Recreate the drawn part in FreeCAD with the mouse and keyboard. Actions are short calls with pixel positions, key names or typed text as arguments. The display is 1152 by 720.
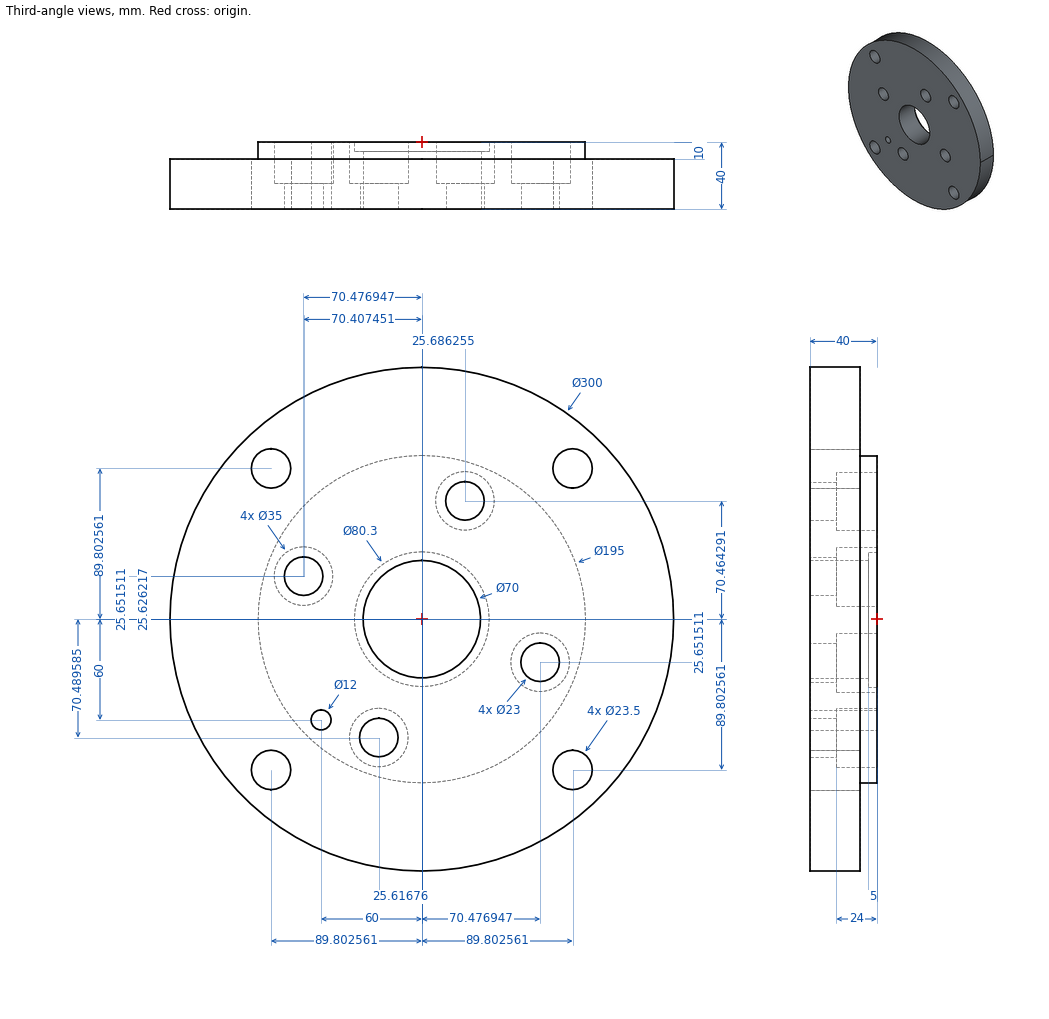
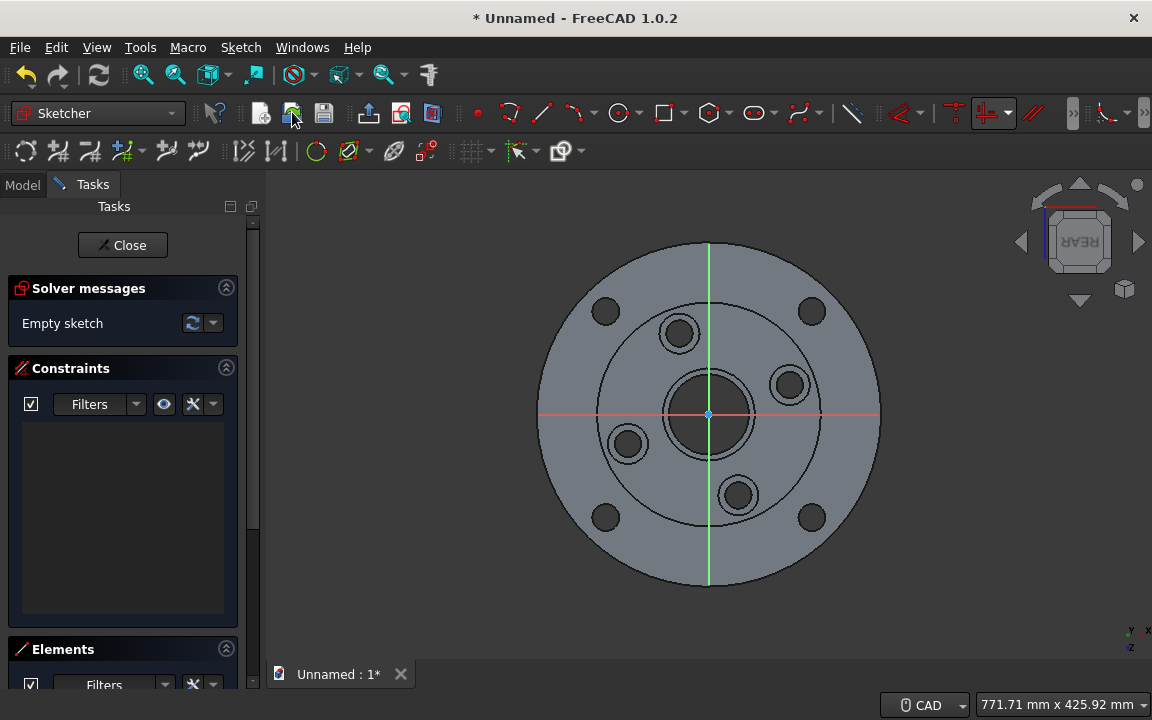
scroll(640, 342, up, 15)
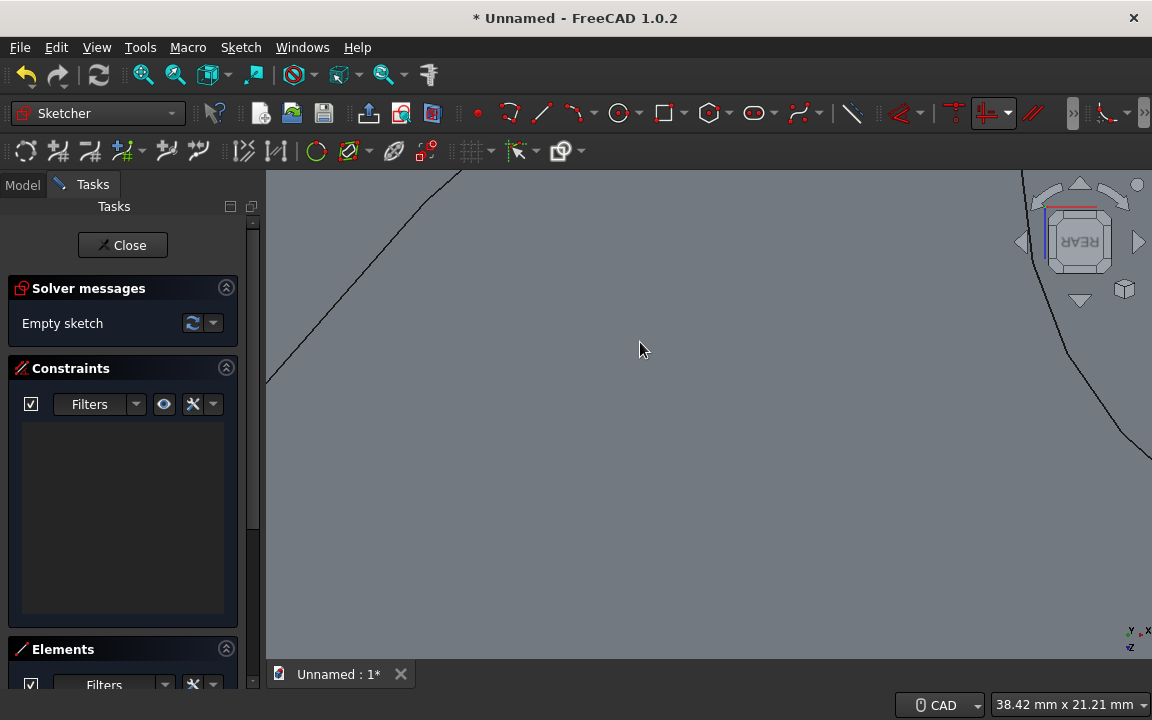
click(620, 114)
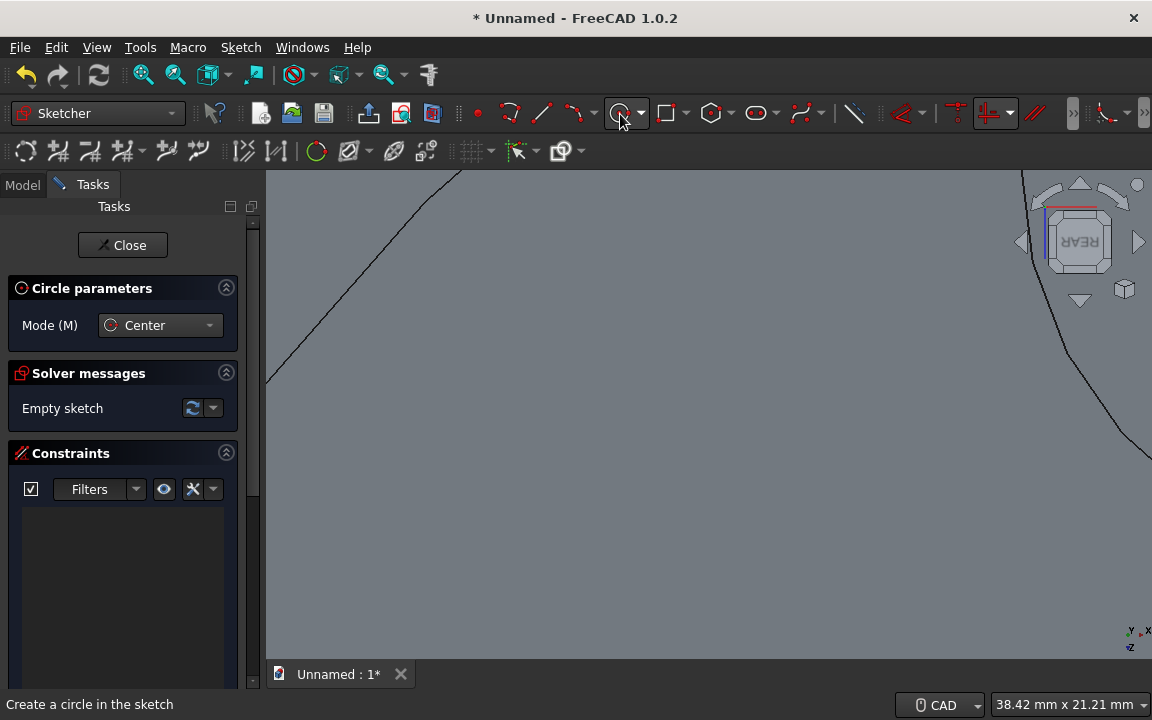
click(632, 408)
move(730, 310)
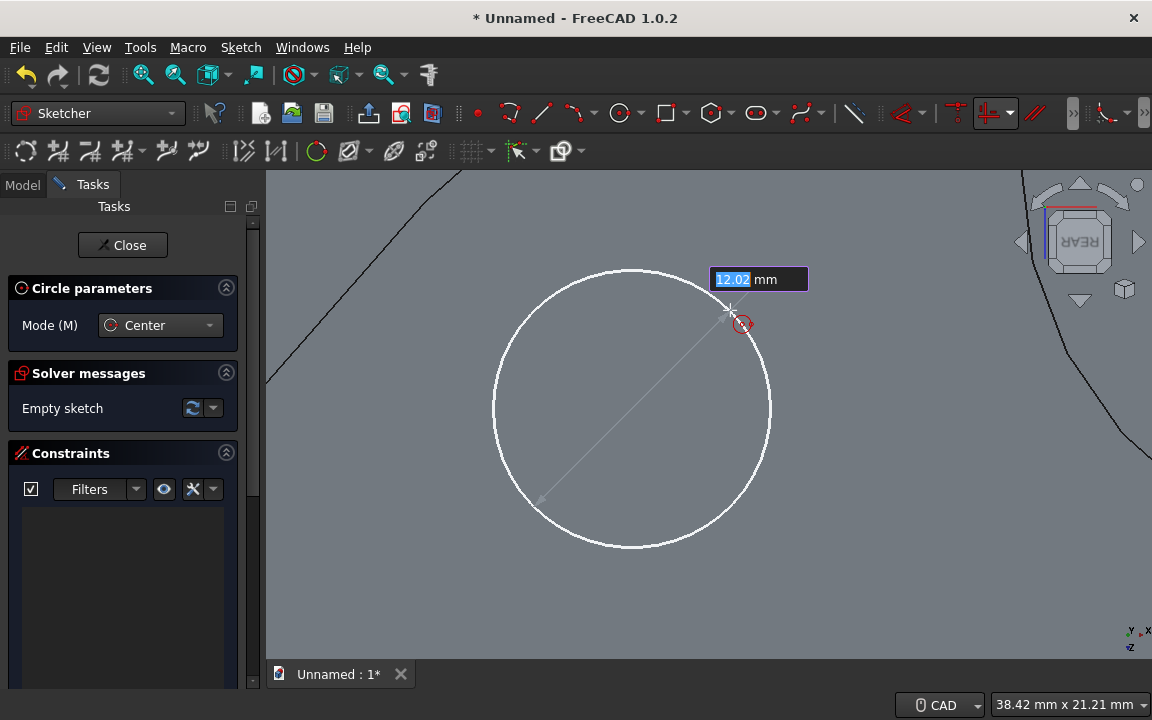
text(12)
key(Return)
key(Escape)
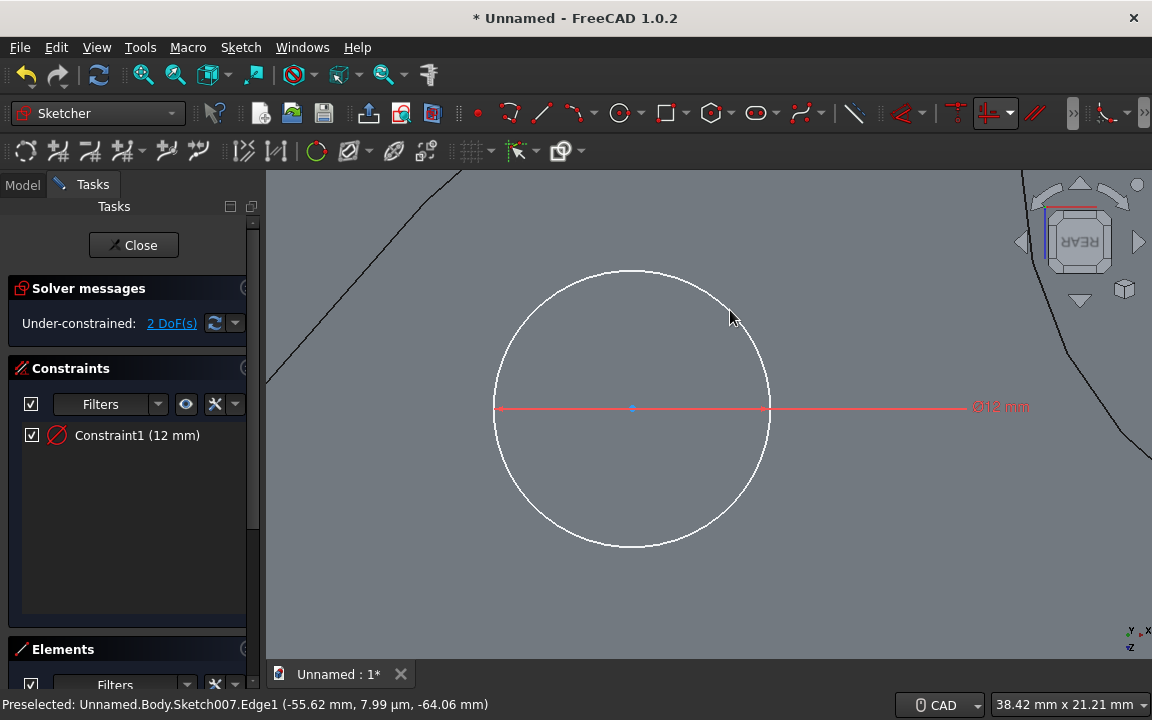
click(902, 114)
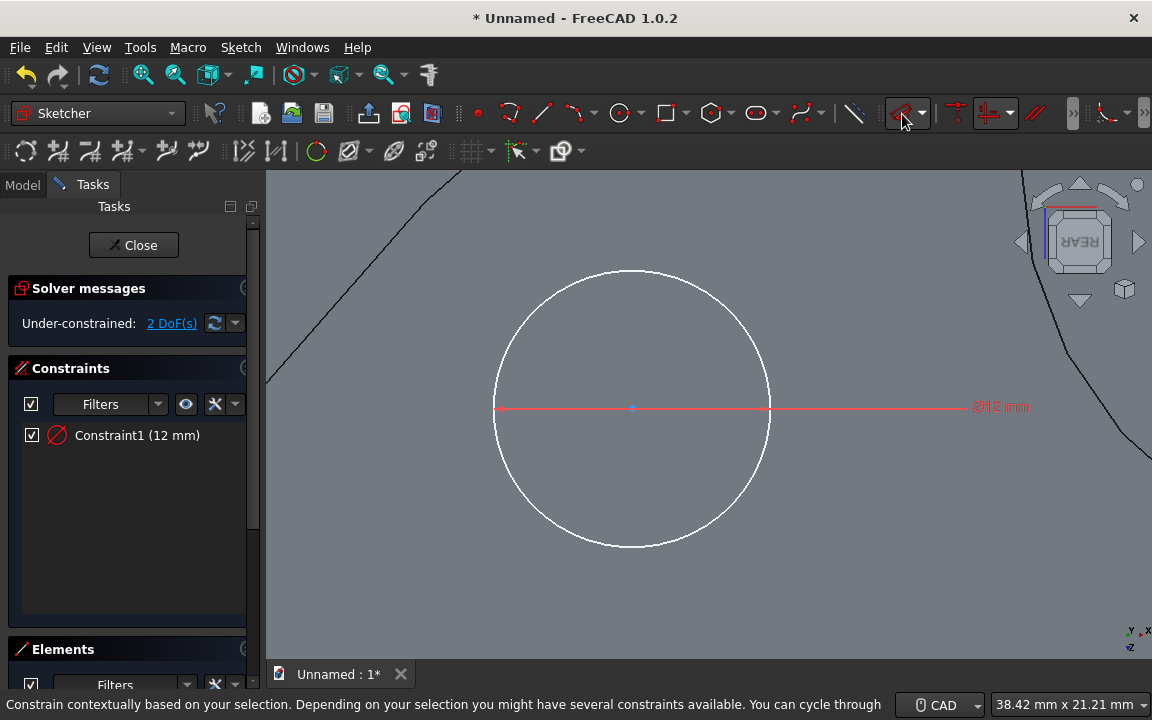
click(632, 409)
click(810, 375)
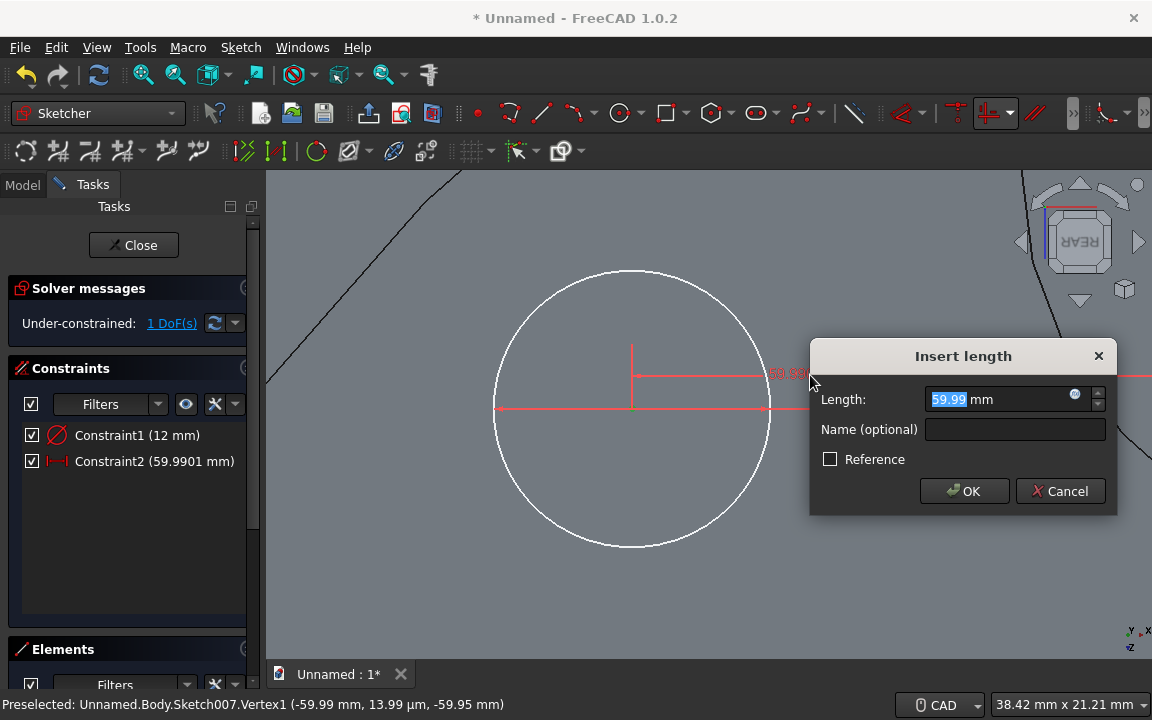
text(60)
key(Return)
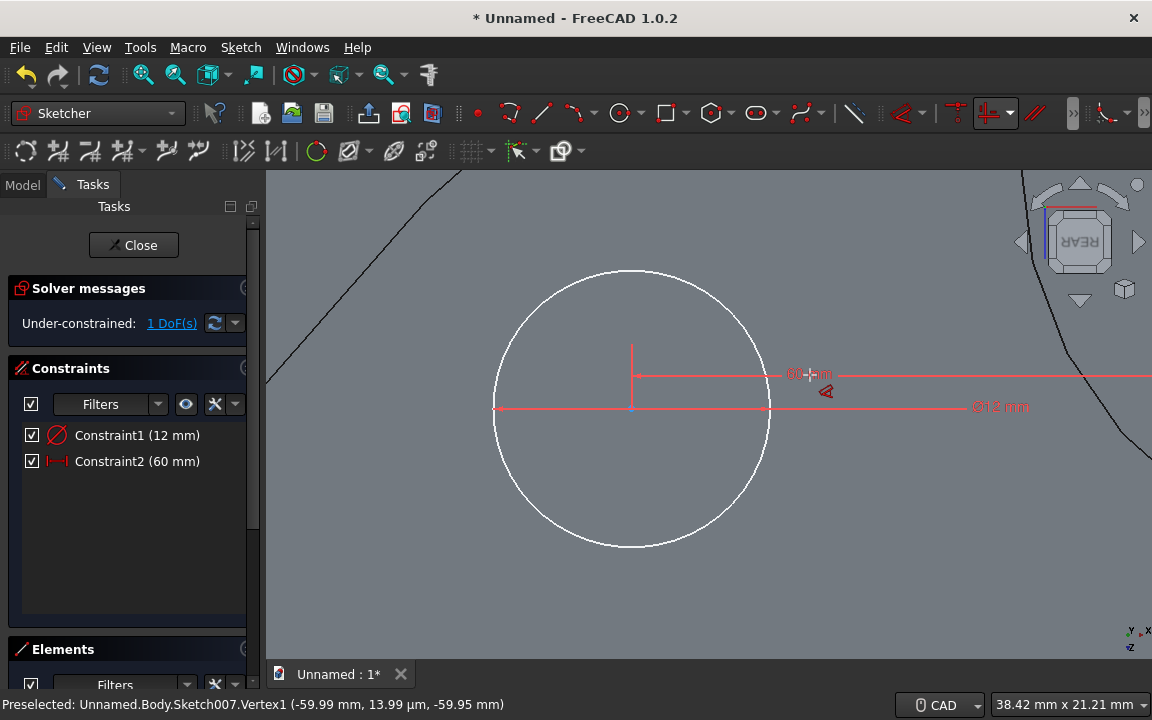
click(632, 409)
click(598, 520)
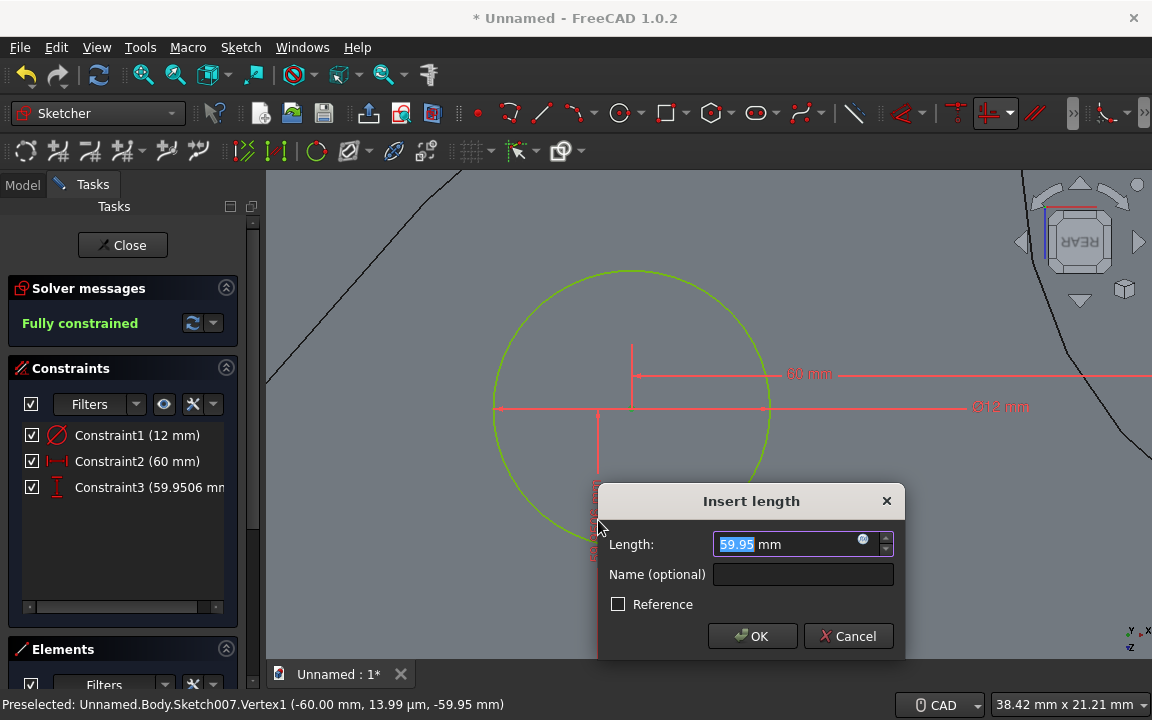
text(60)
key(Return)
key(Escape)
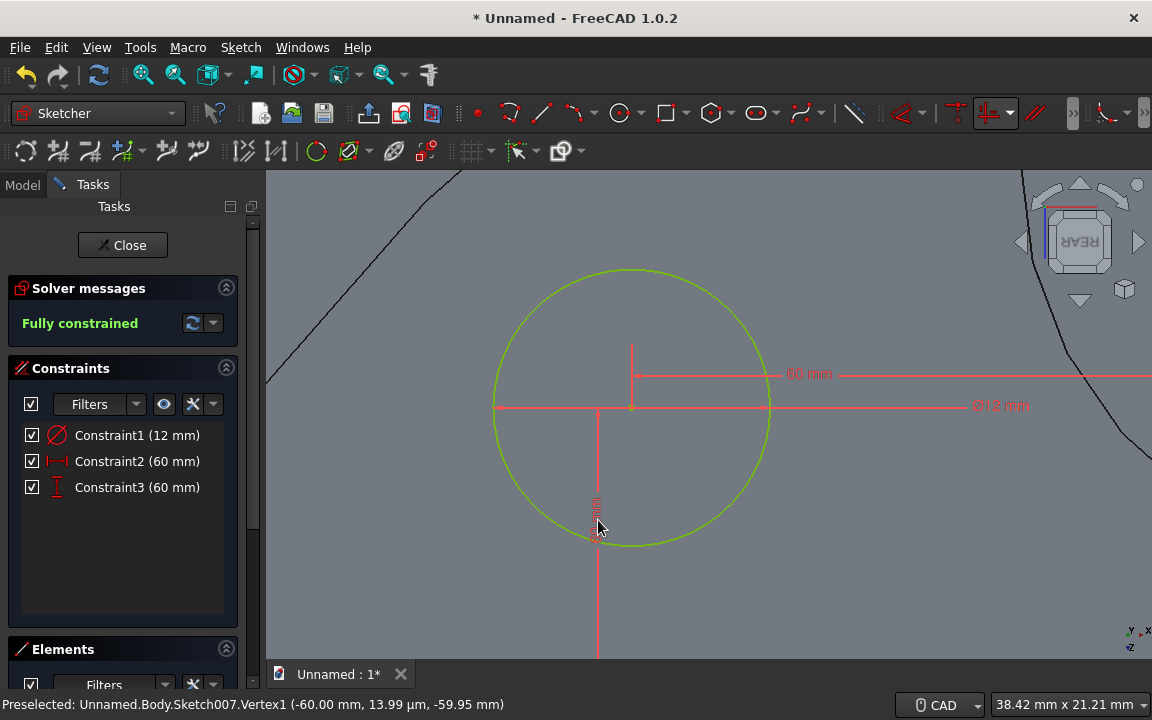
click(123, 245)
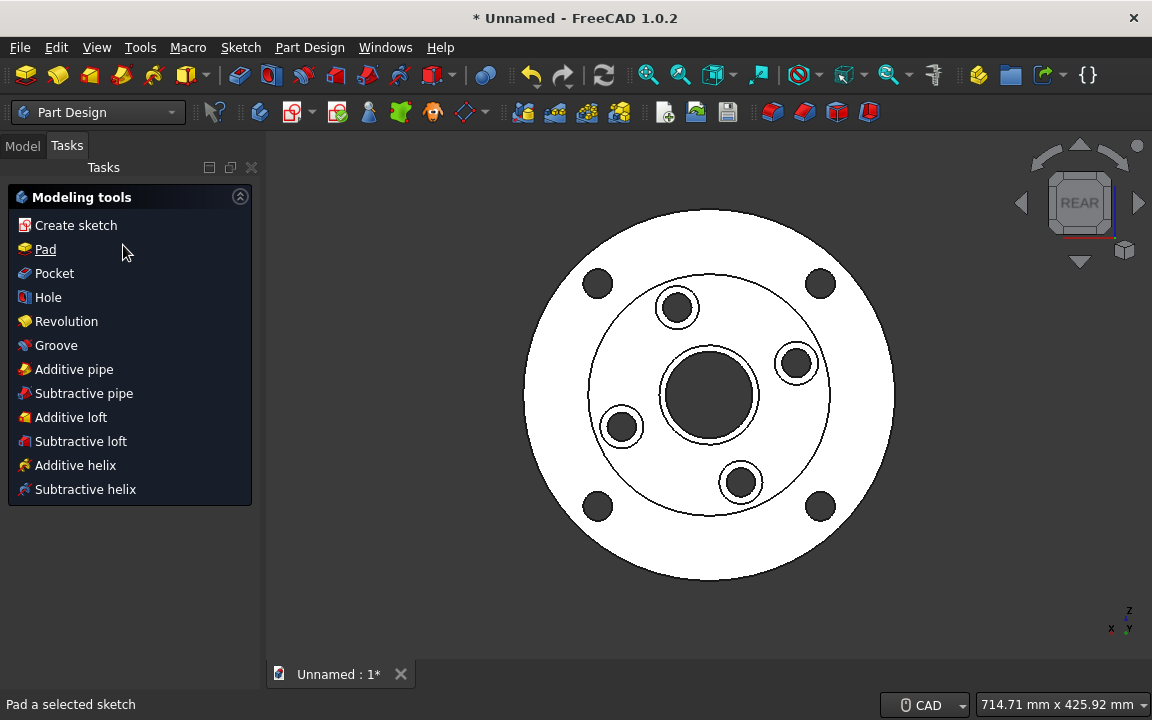
click(240, 76)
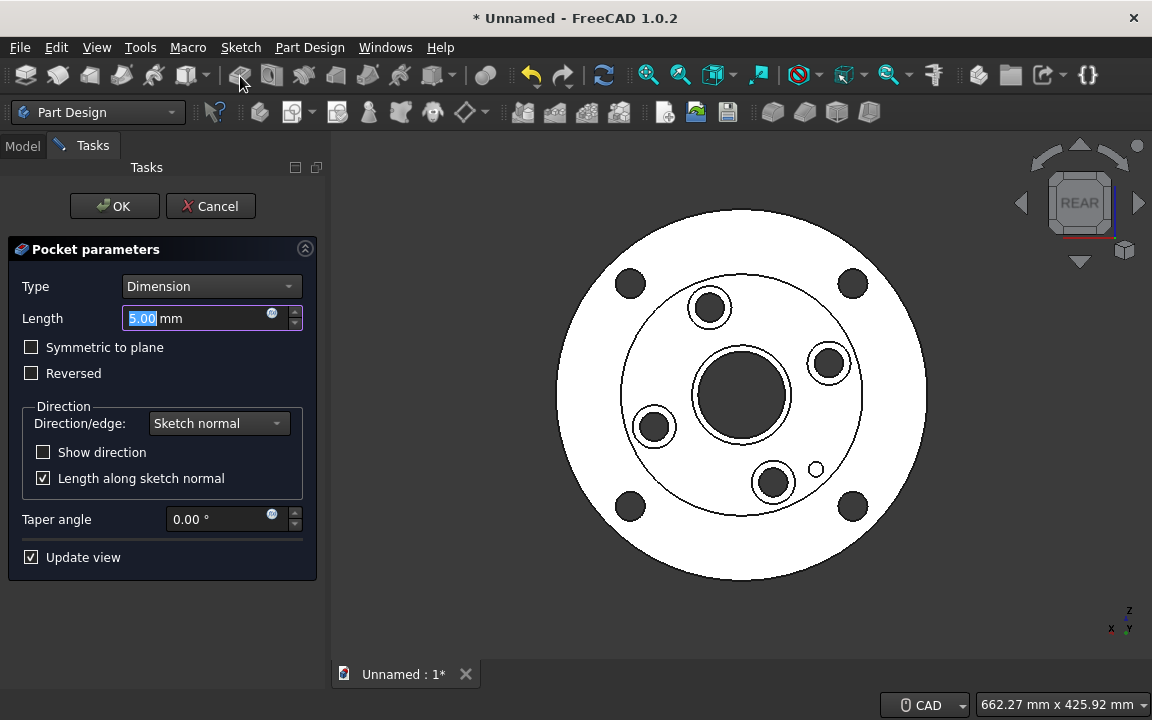
click(212, 286)